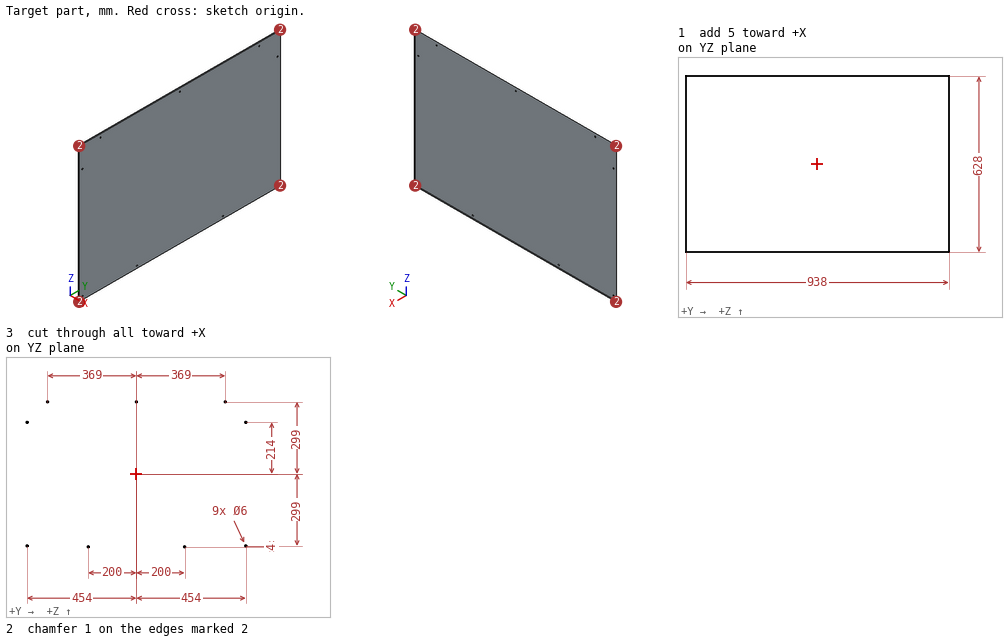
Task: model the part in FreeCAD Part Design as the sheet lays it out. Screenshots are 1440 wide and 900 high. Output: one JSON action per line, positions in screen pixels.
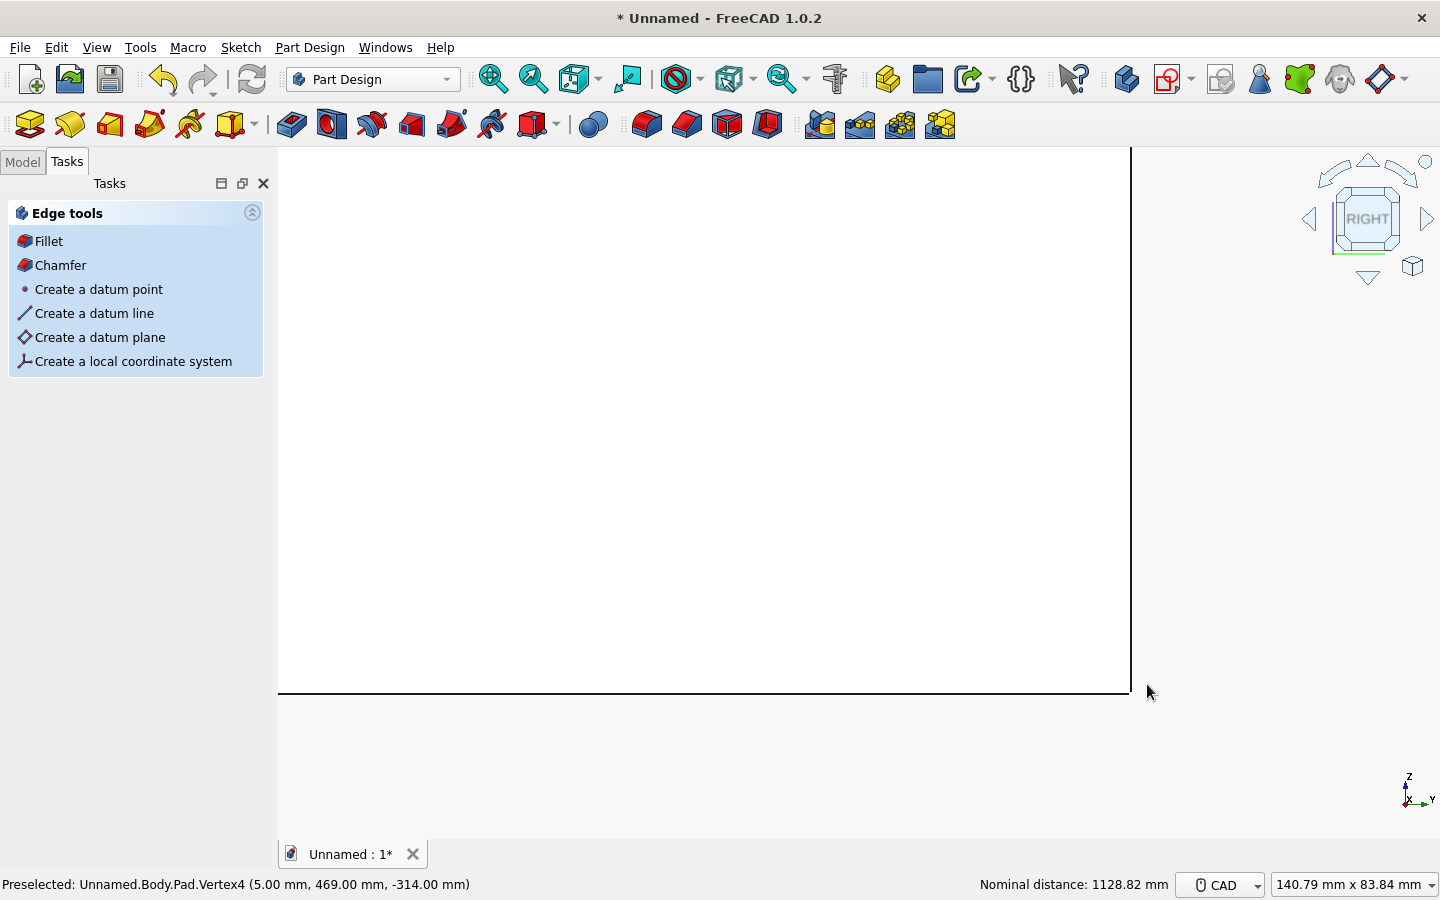
{"action": "key", "text": "v f"}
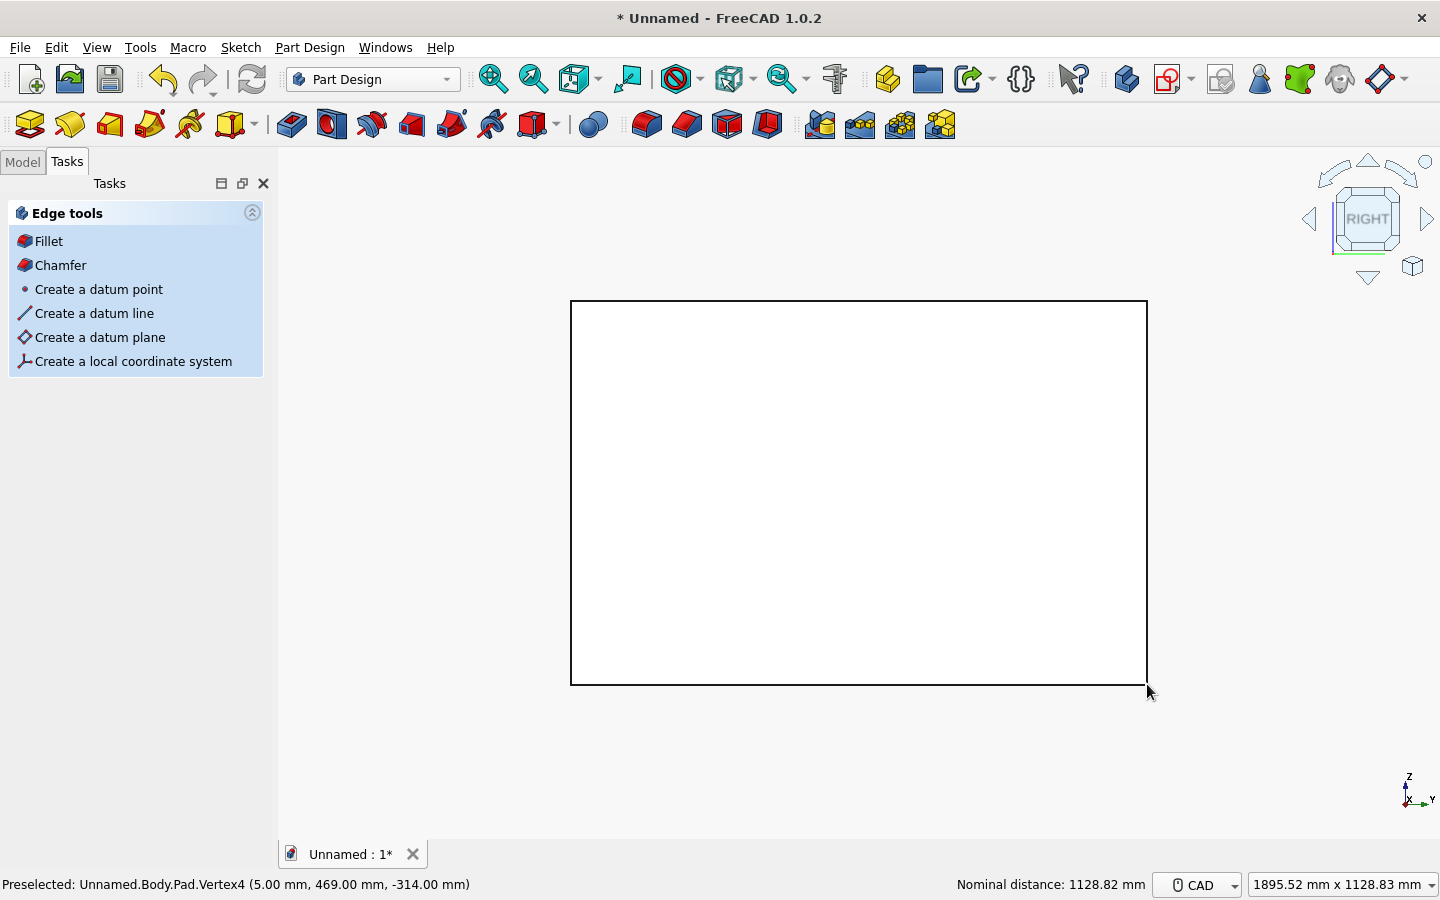
{"action": "key", "text": "5"}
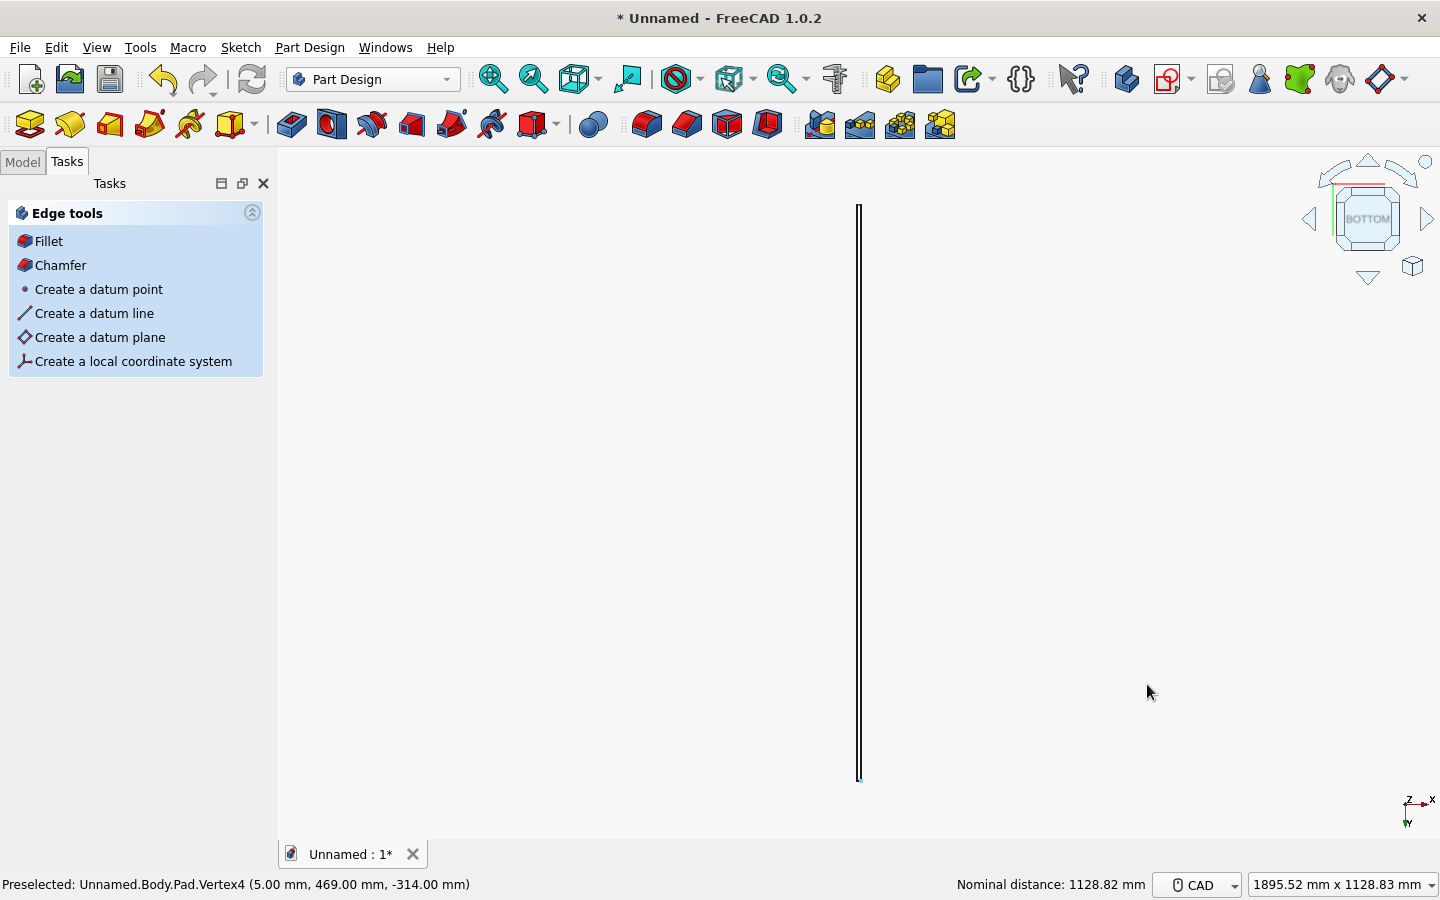
{"action": "scroll", "coordinate": [859, 780], "scroll_direction": "up", "scroll_amount": 13}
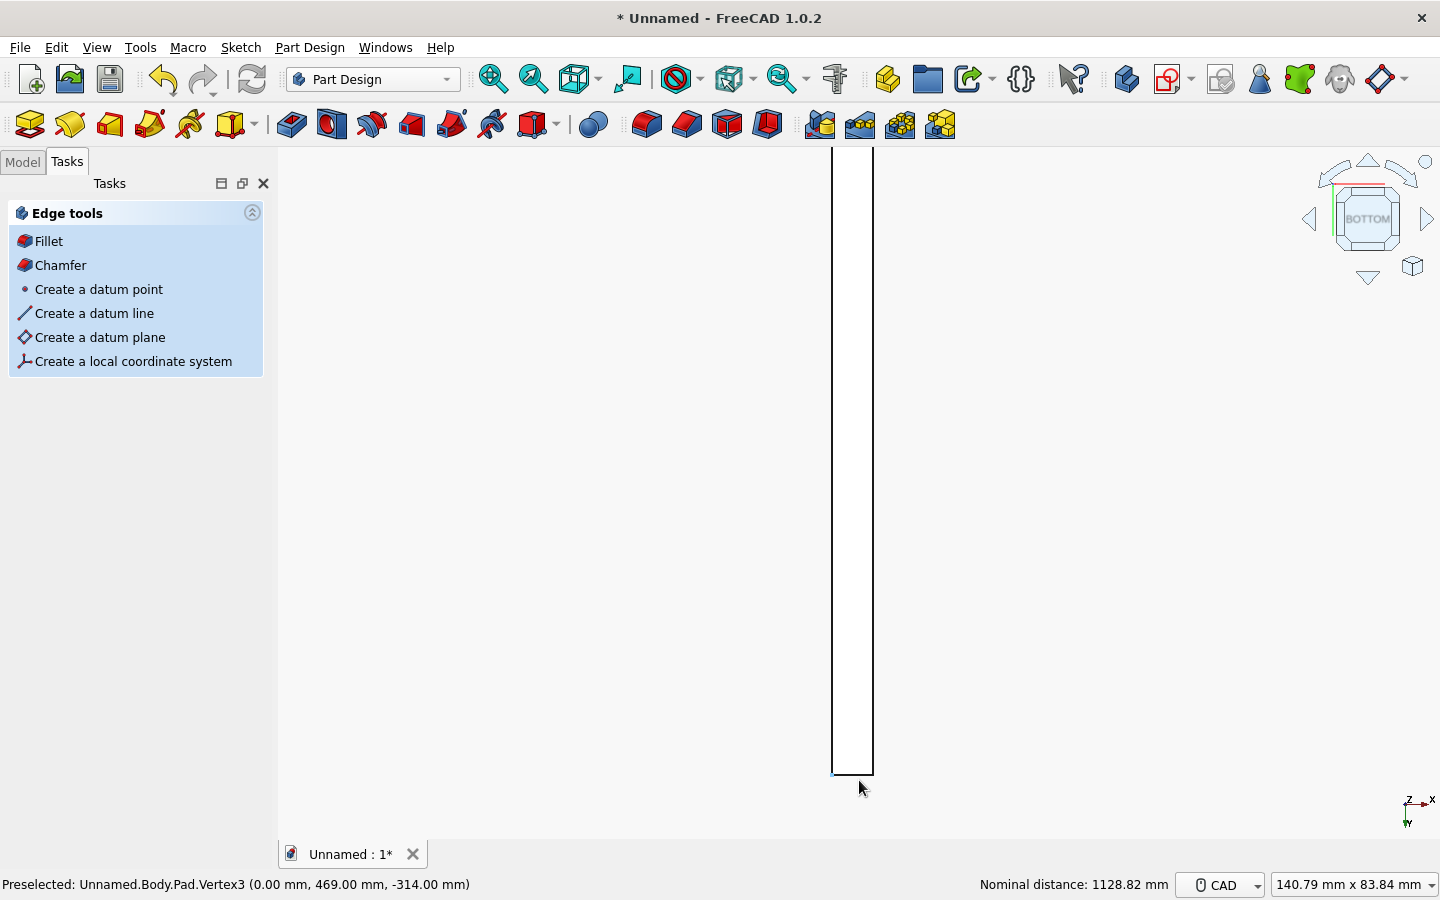
{"action": "left_click", "coordinate": [853, 774], "text": "ctrl"}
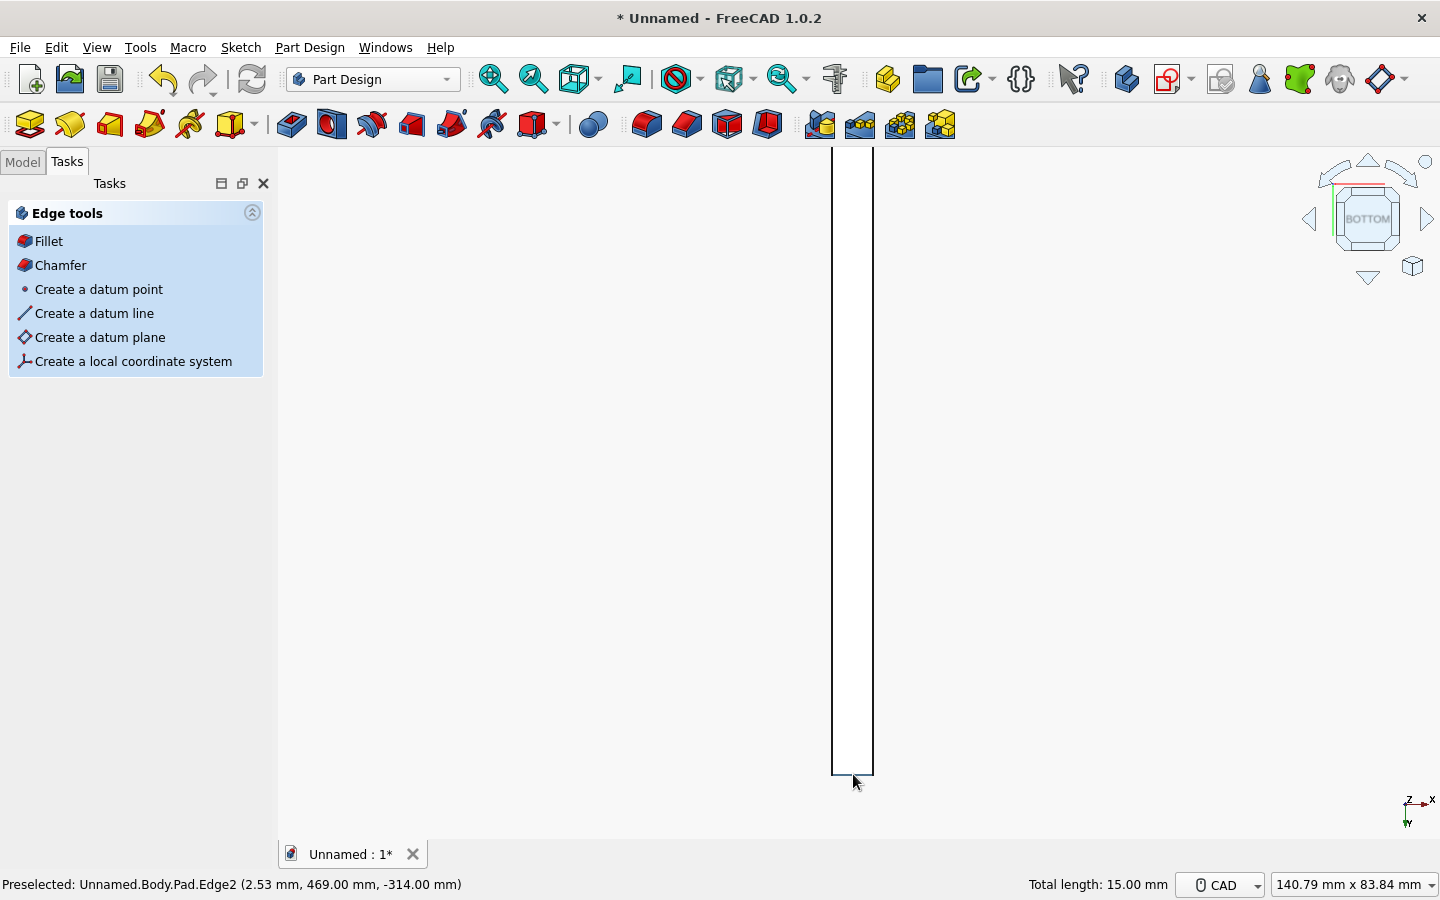
{"action": "key", "text": "v f"}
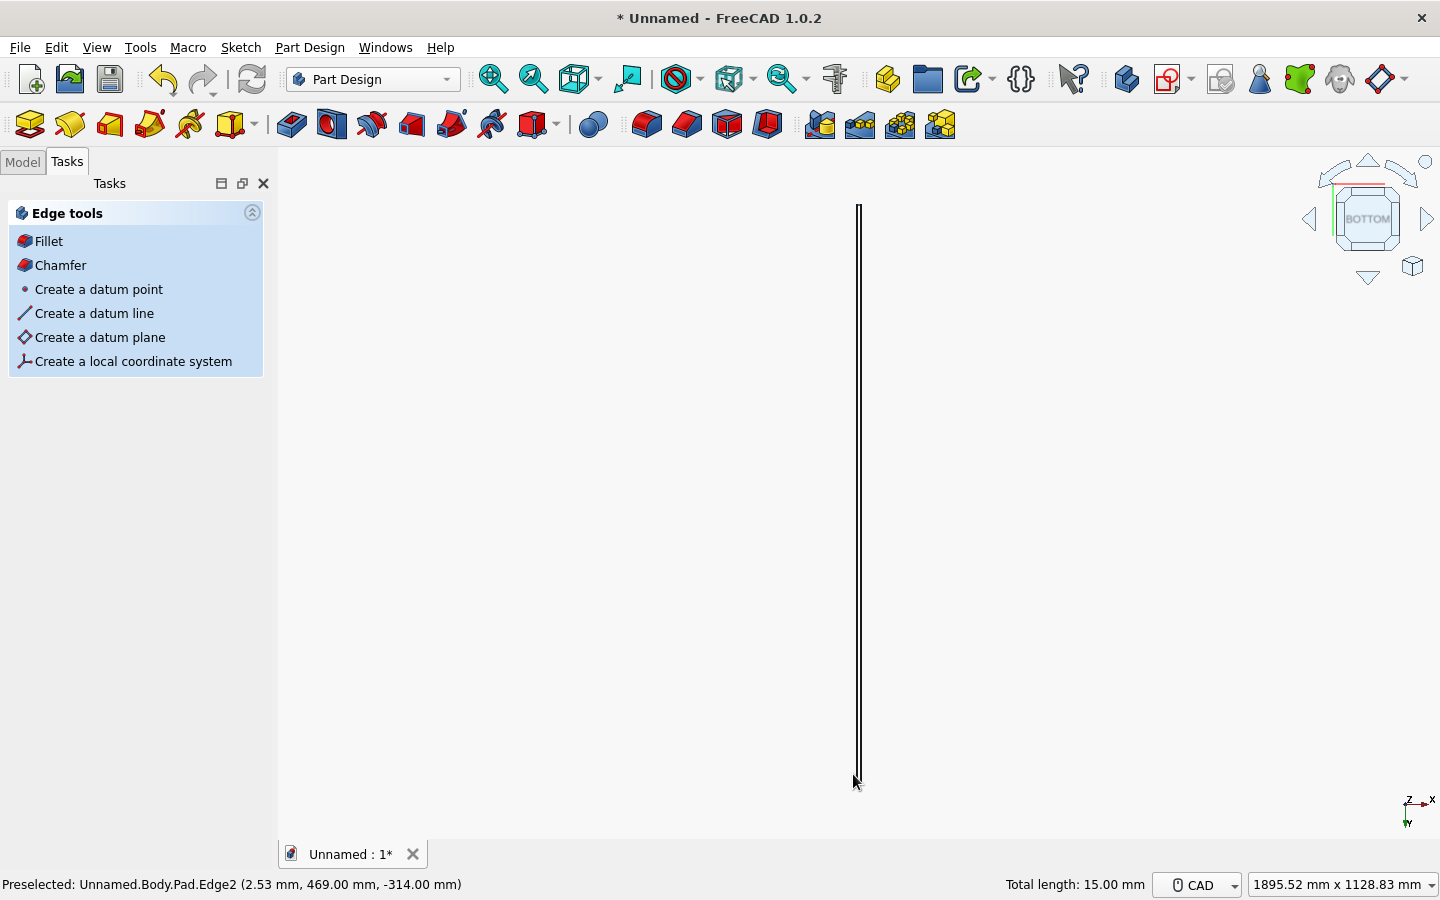
{"action": "key", "text": "4"}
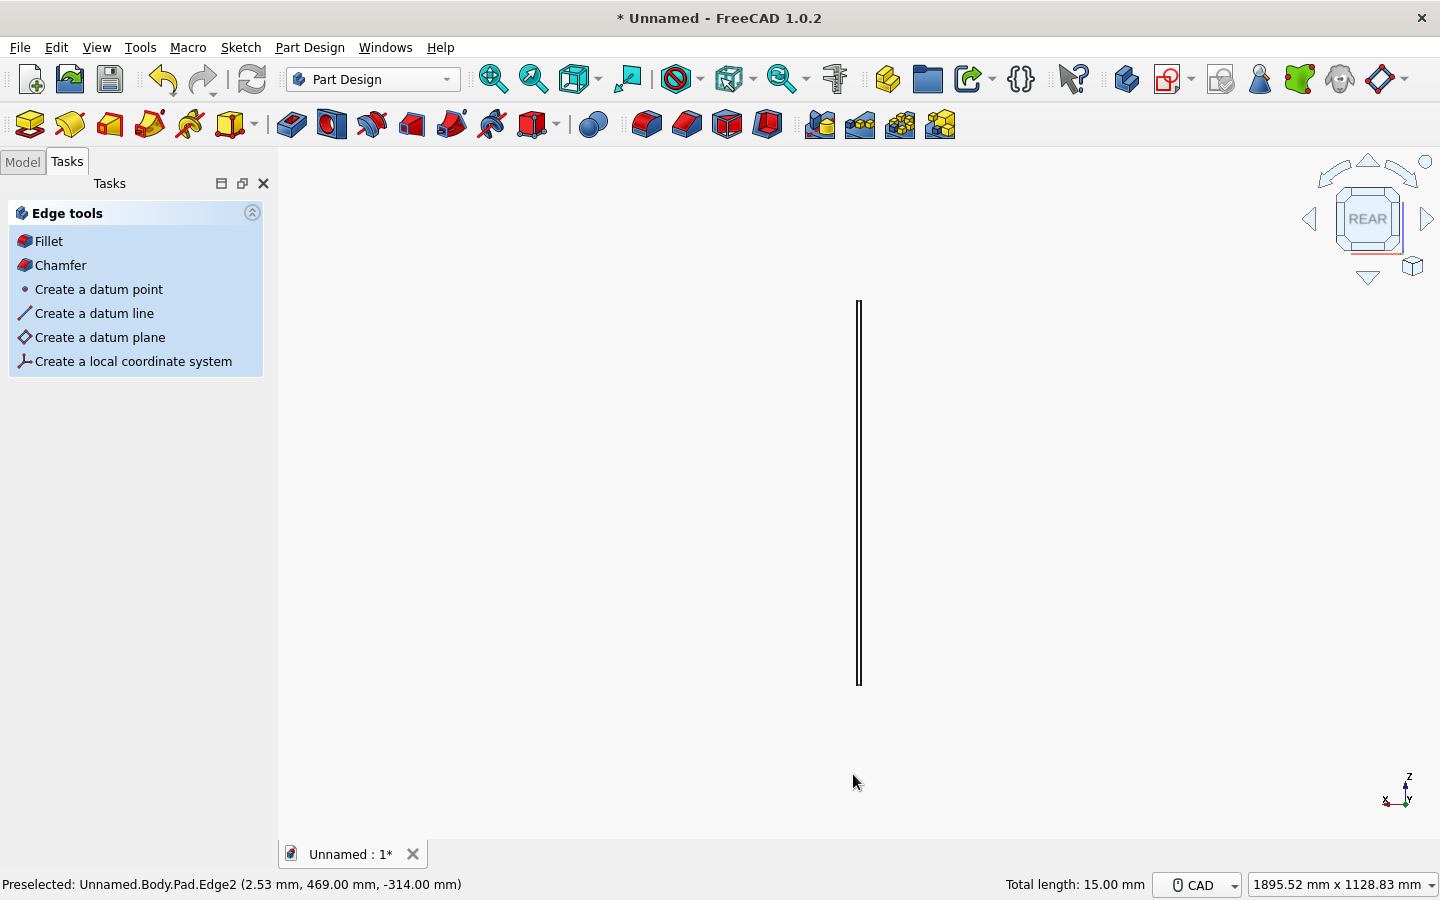
{"action": "scroll", "coordinate": [859, 300], "scroll_direction": "up", "scroll_amount": 13}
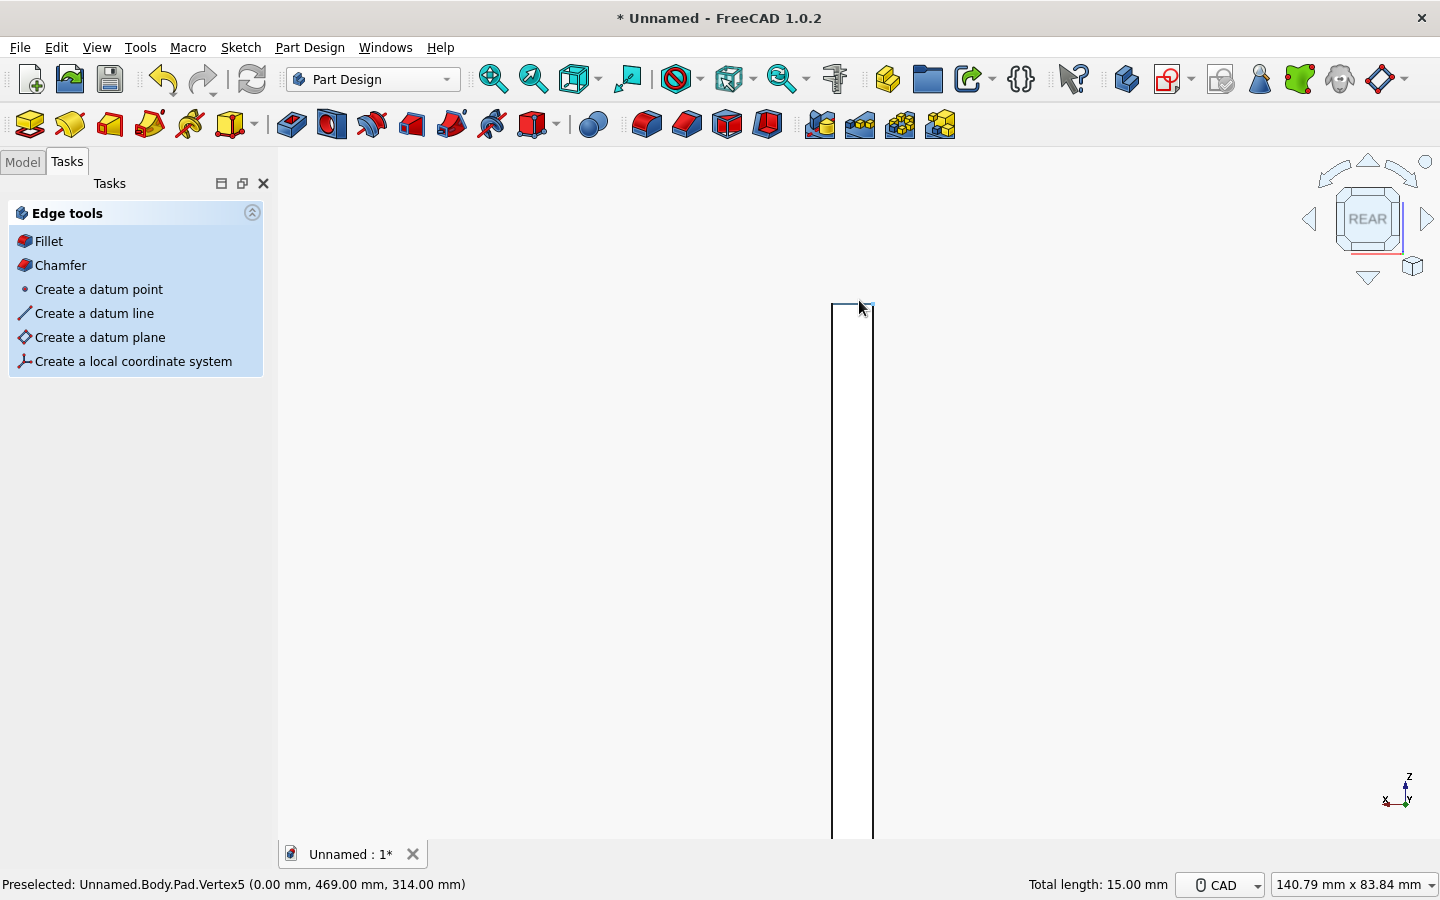
{"action": "key", "text": "v f"}